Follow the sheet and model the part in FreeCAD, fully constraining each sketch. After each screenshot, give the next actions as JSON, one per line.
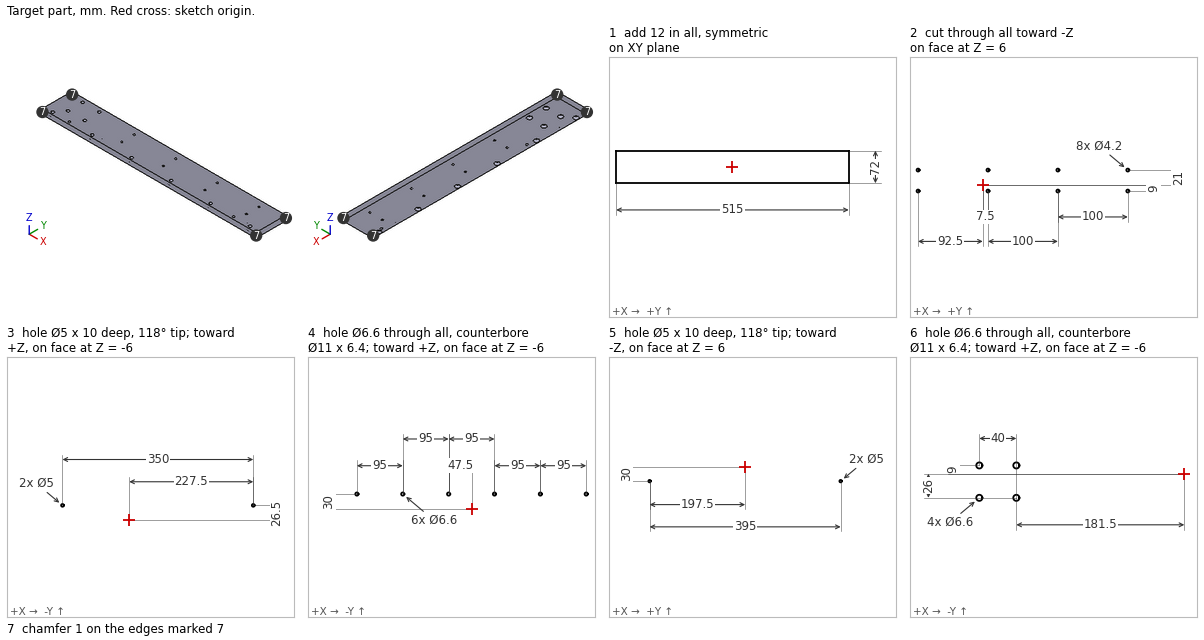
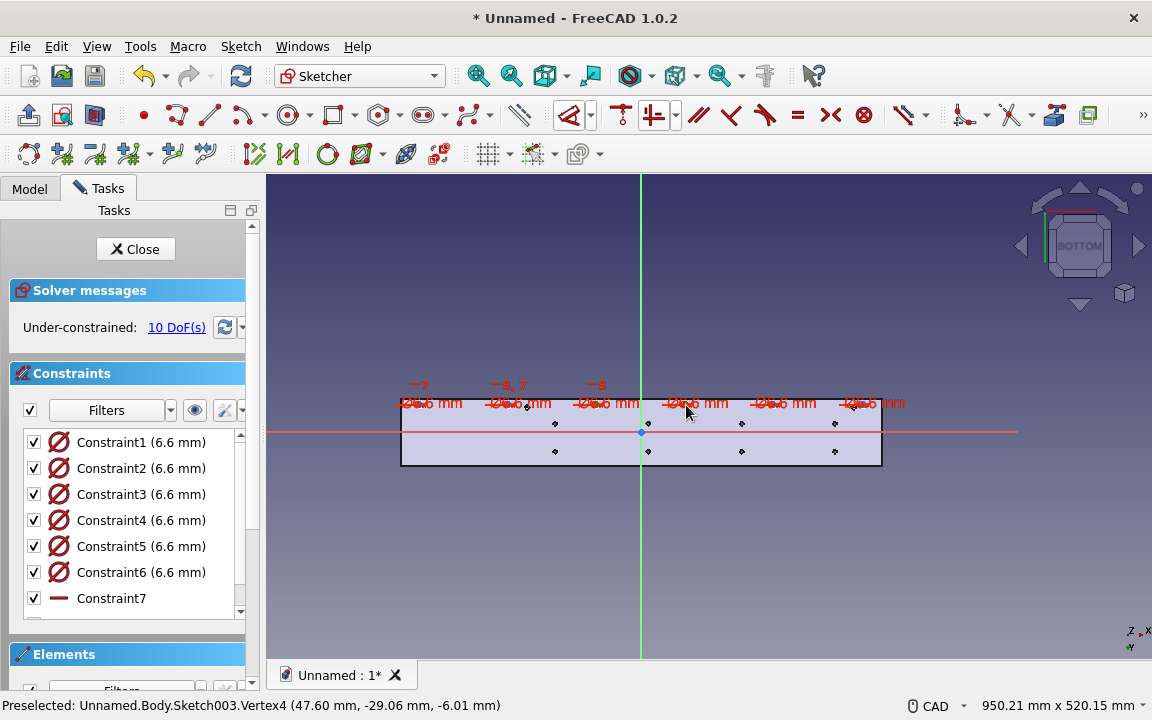
{"action": "key", "text": "h"}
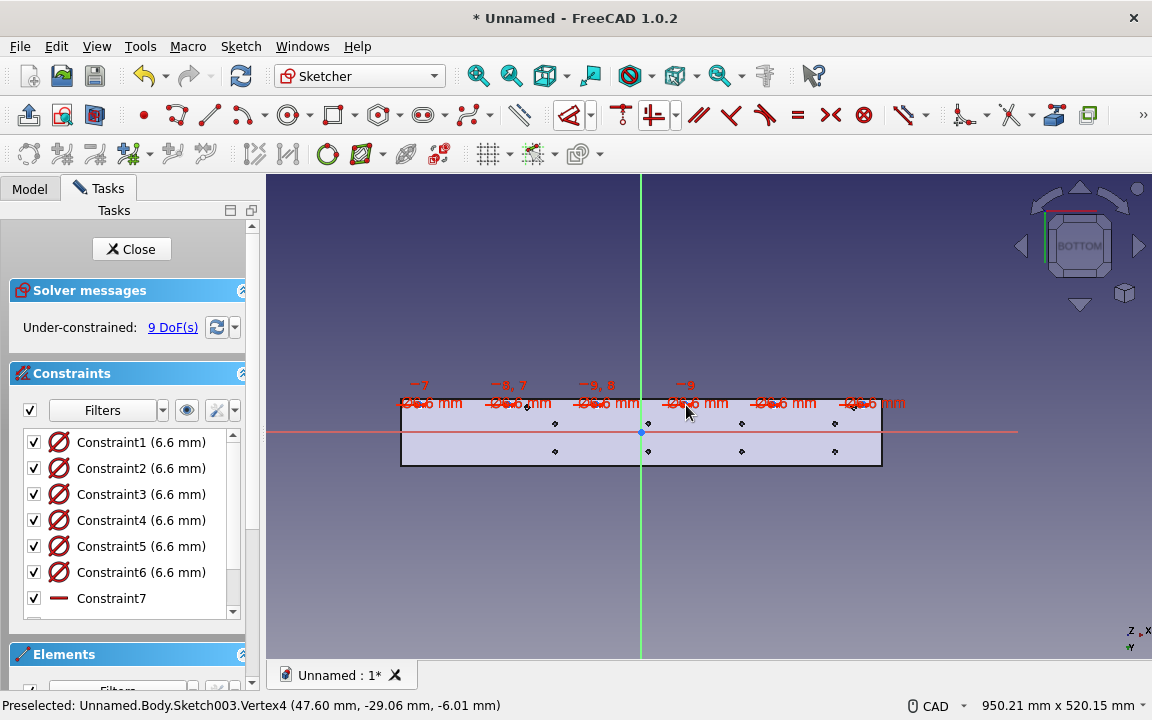
{"action": "left_click", "coordinate": [686, 405]}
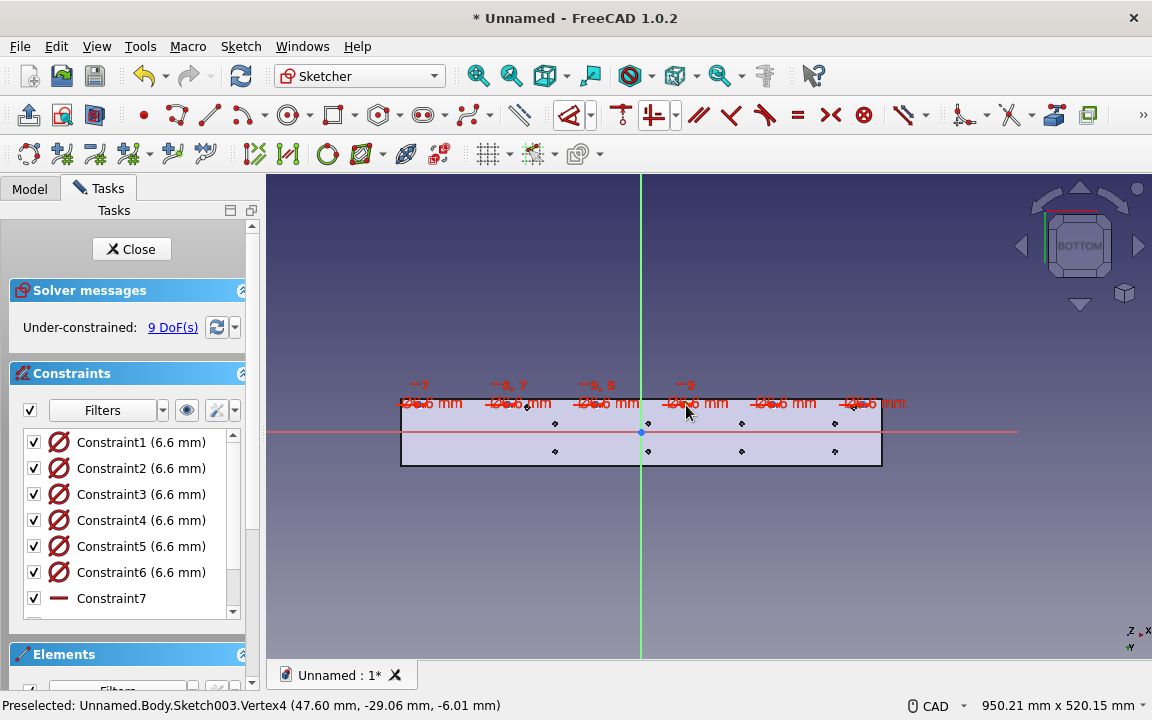
{"action": "left_click", "coordinate": [774, 405]}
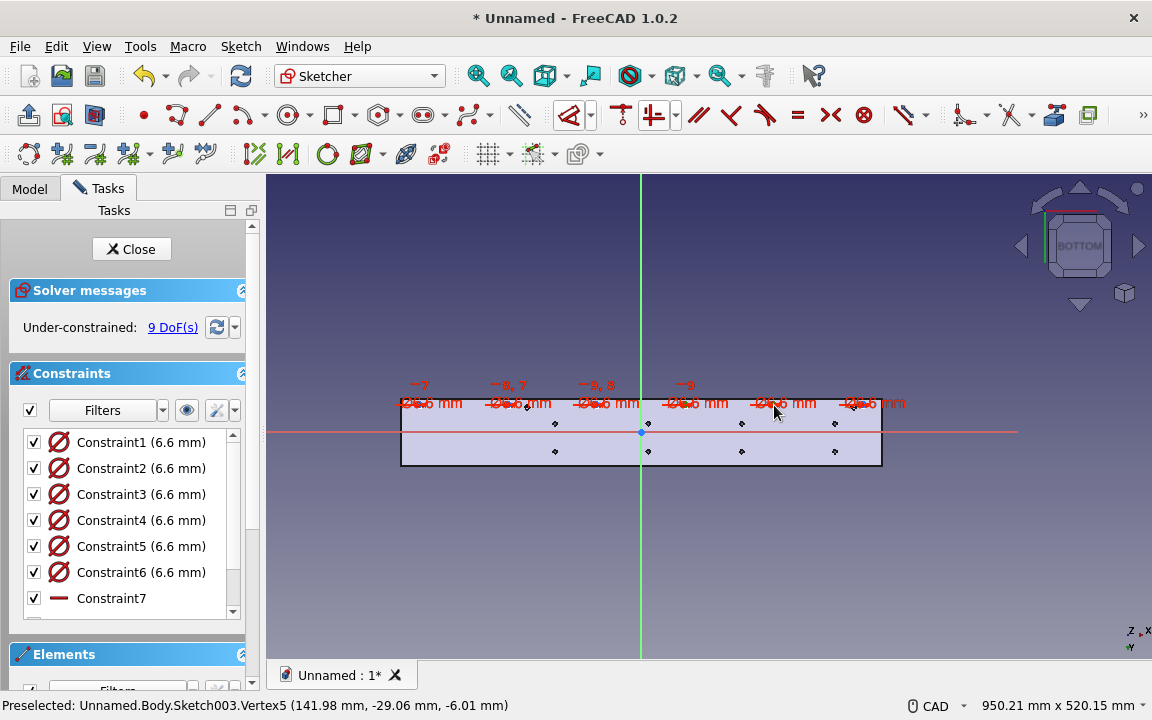
{"action": "left_click", "coordinate": [676, 116]}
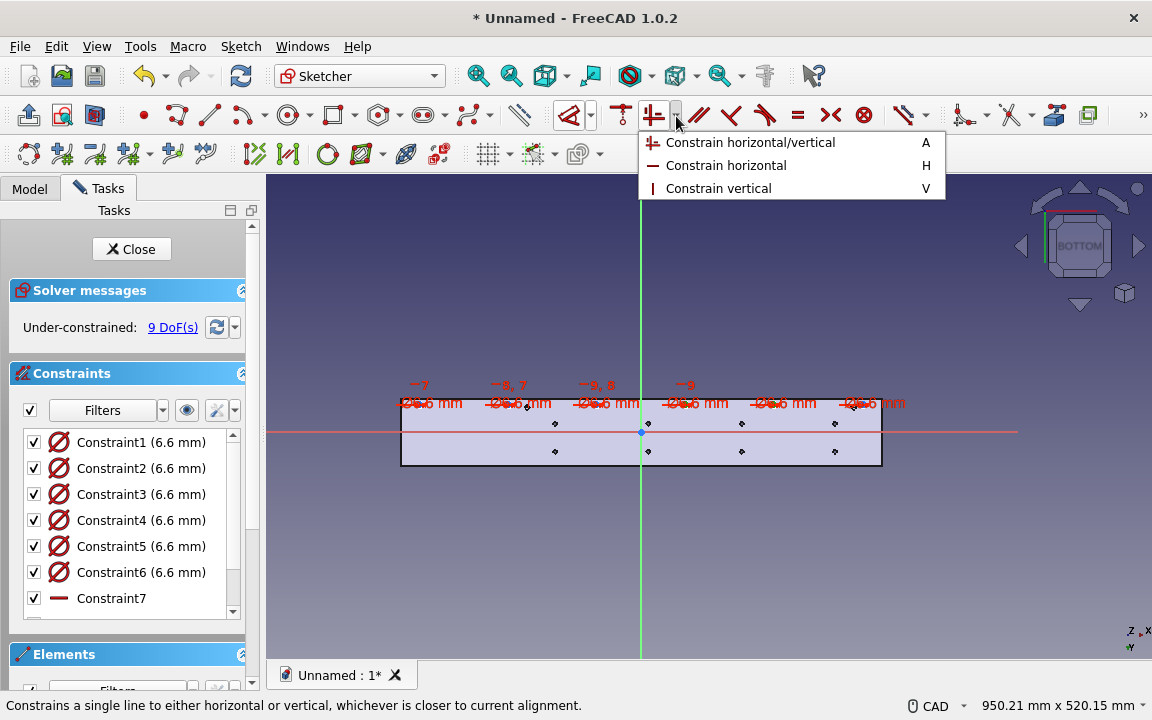
{"action": "left_click", "coordinate": [792, 166]}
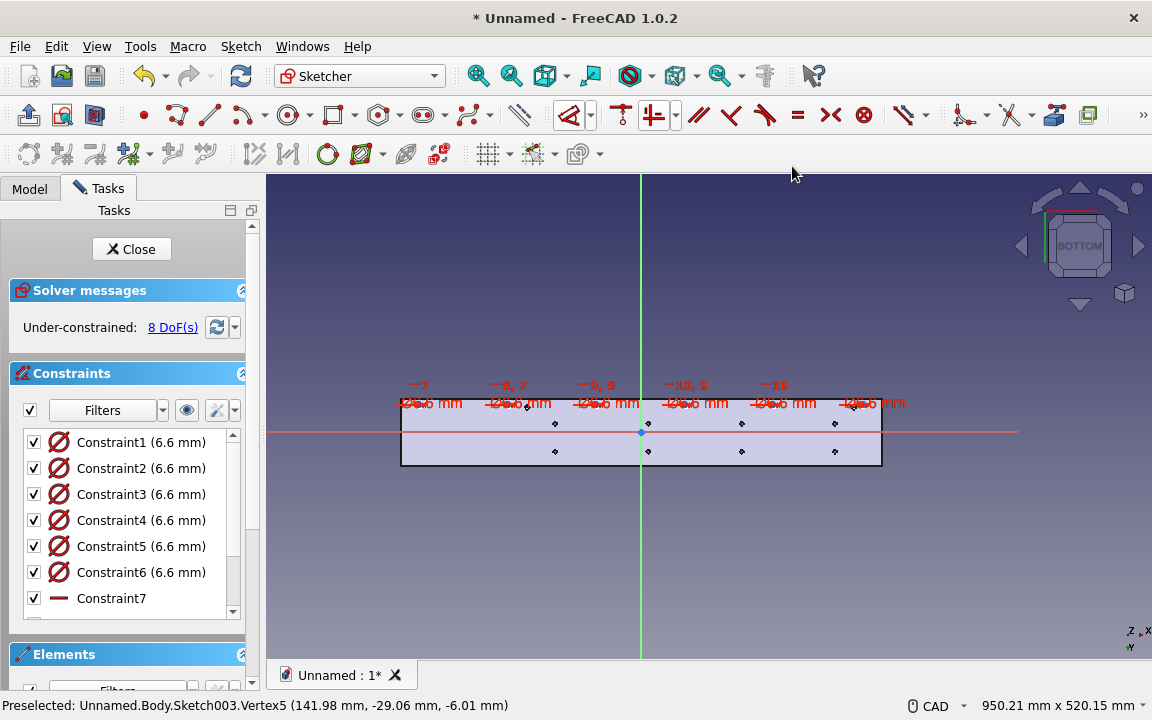
{"action": "left_click", "coordinate": [774, 405]}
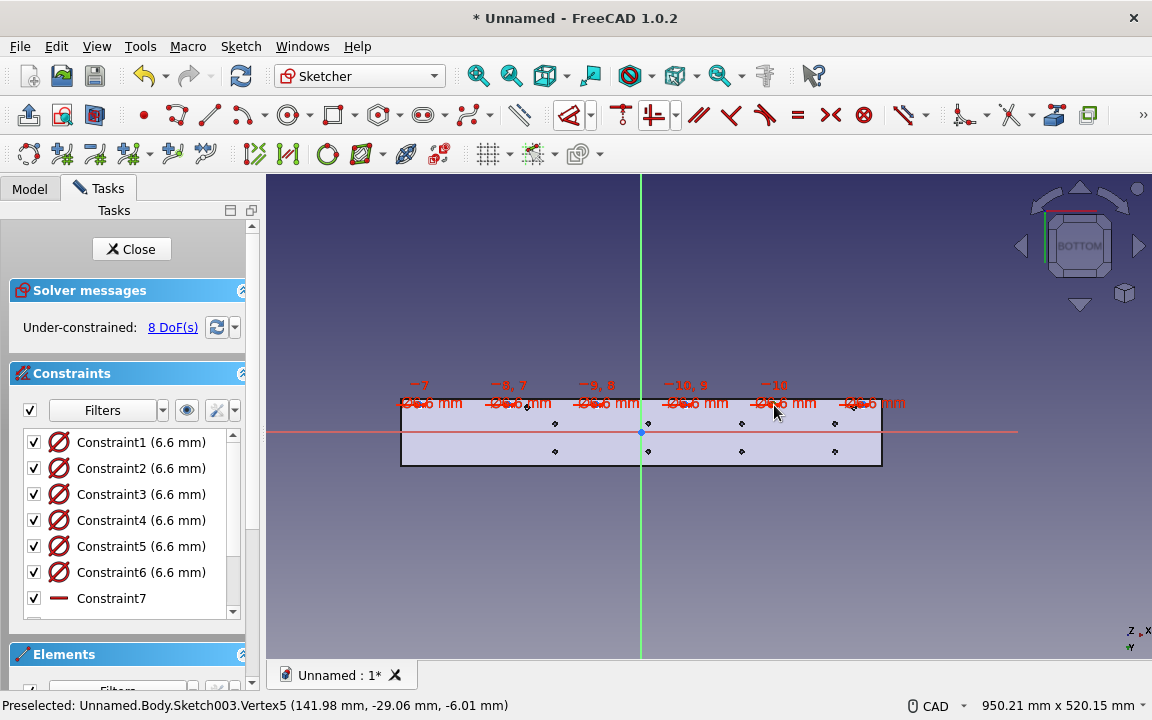
{"action": "left_click", "coordinate": [863, 405]}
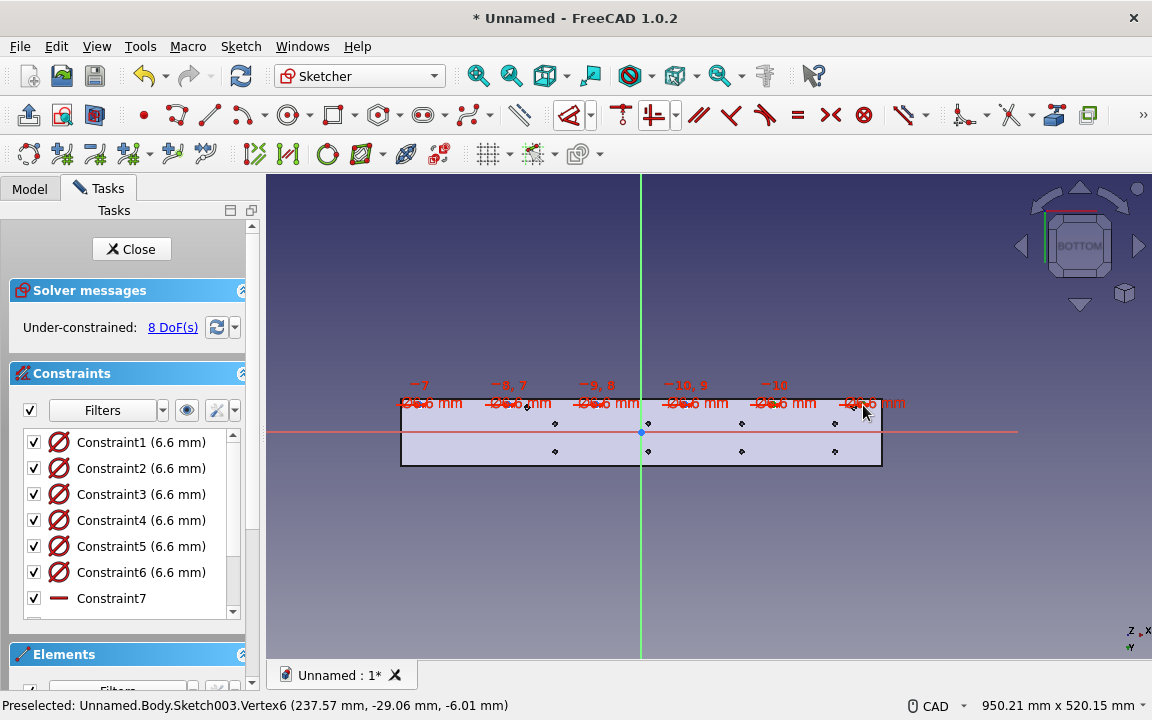
{"action": "left_click", "coordinate": [676, 116]}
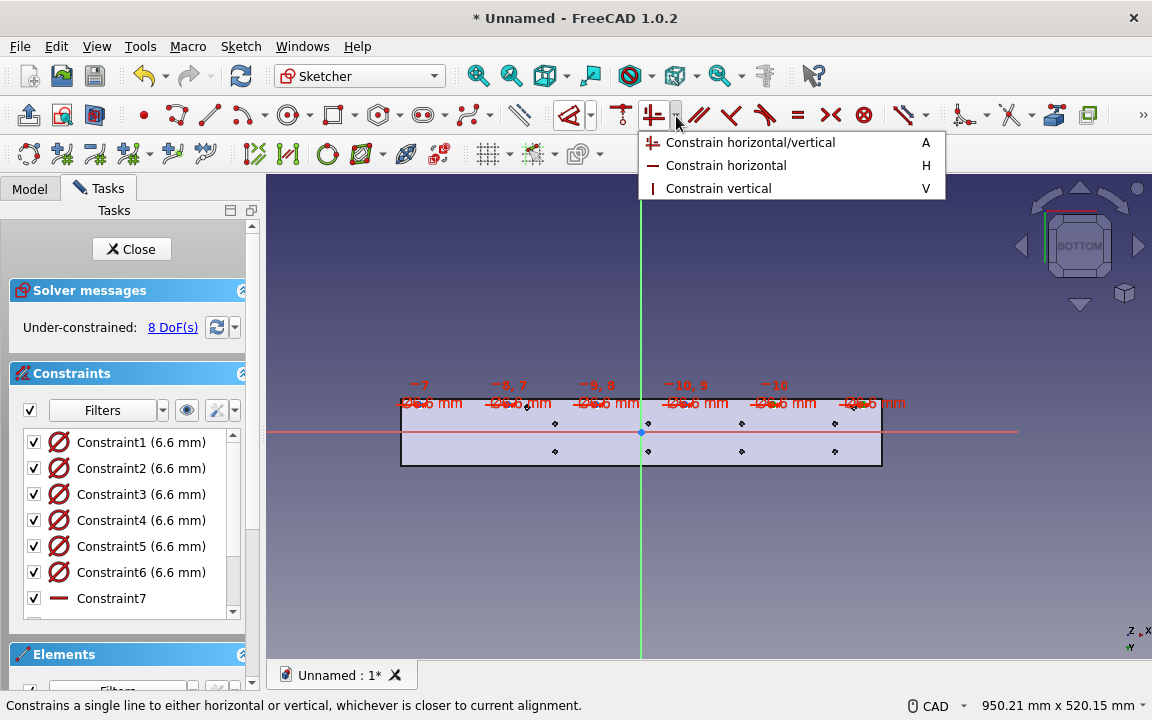
{"action": "left_click", "coordinate": [792, 166]}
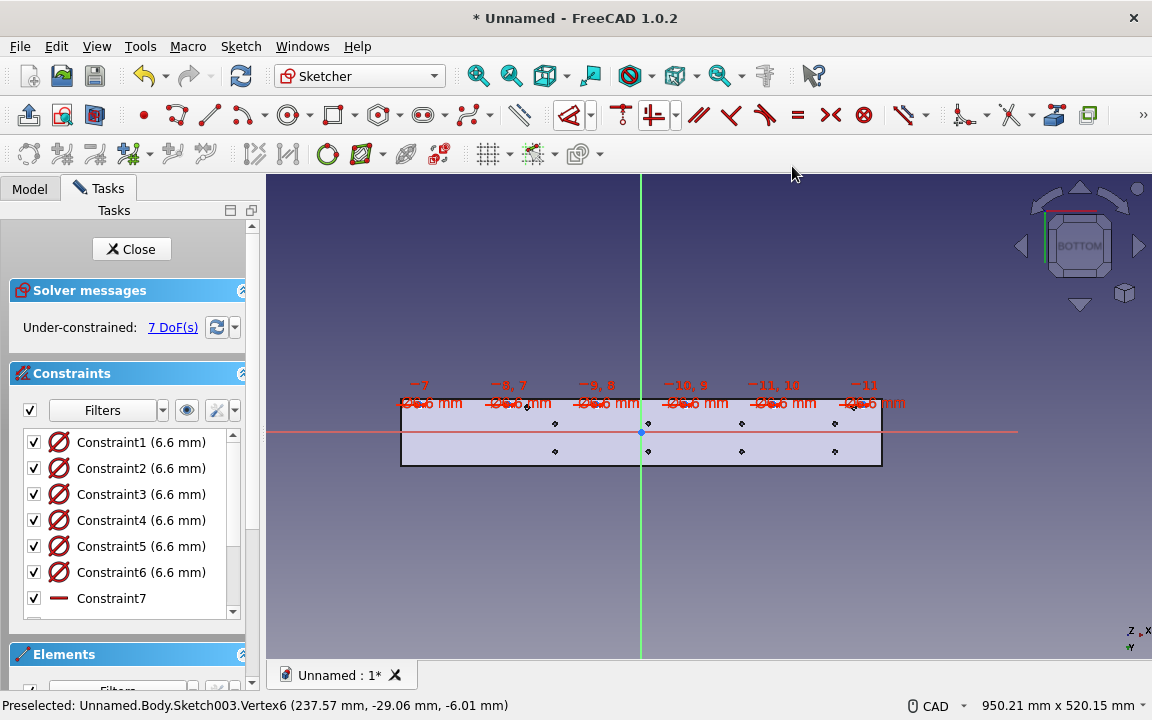
{"action": "scroll", "coordinate": [420, 405], "scroll_direction": "up", "scroll_amount": 2}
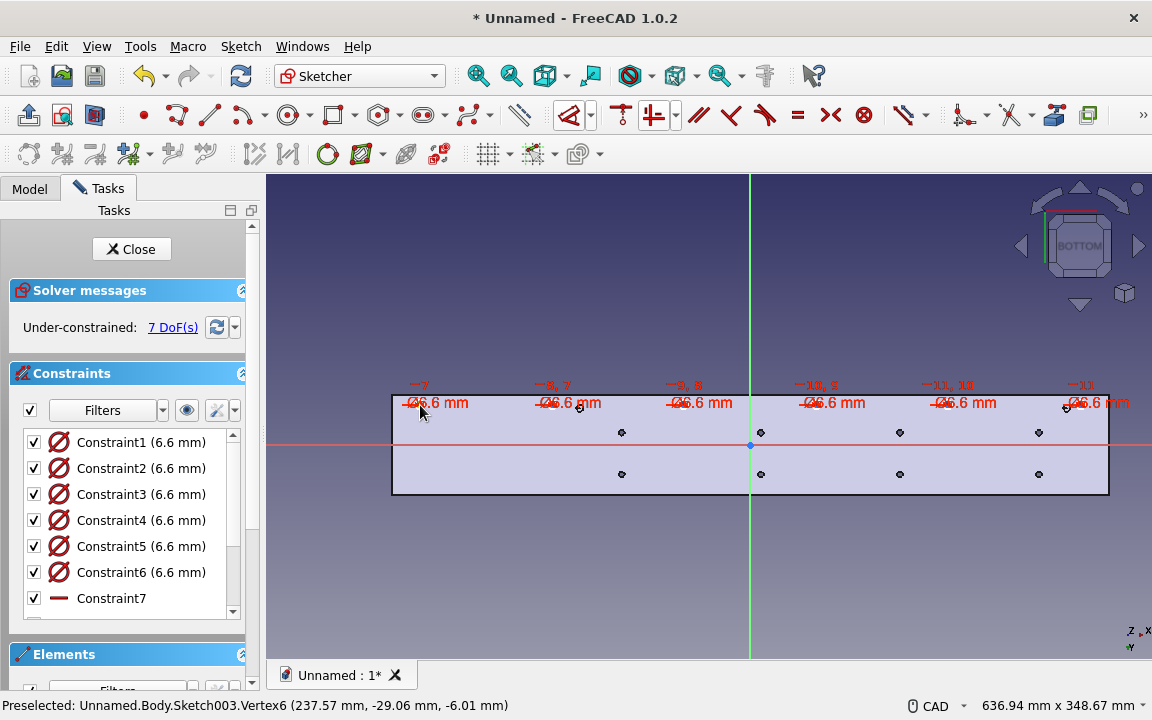
{"action": "left_click", "coordinate": [420, 405]}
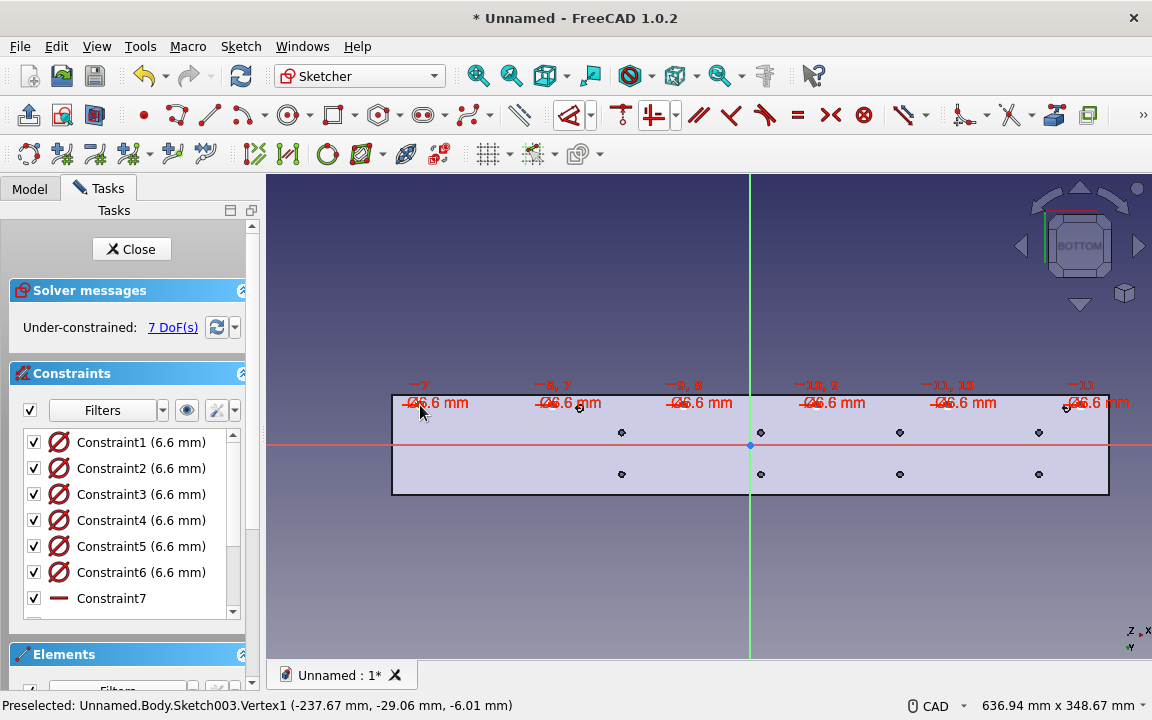
{"action": "left_click", "coordinate": [590, 116]}